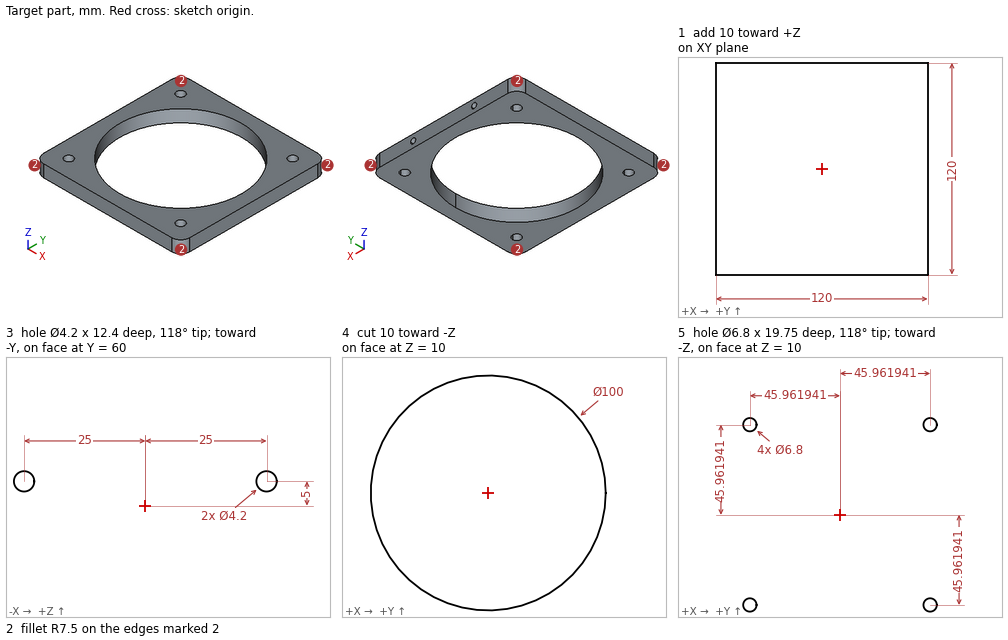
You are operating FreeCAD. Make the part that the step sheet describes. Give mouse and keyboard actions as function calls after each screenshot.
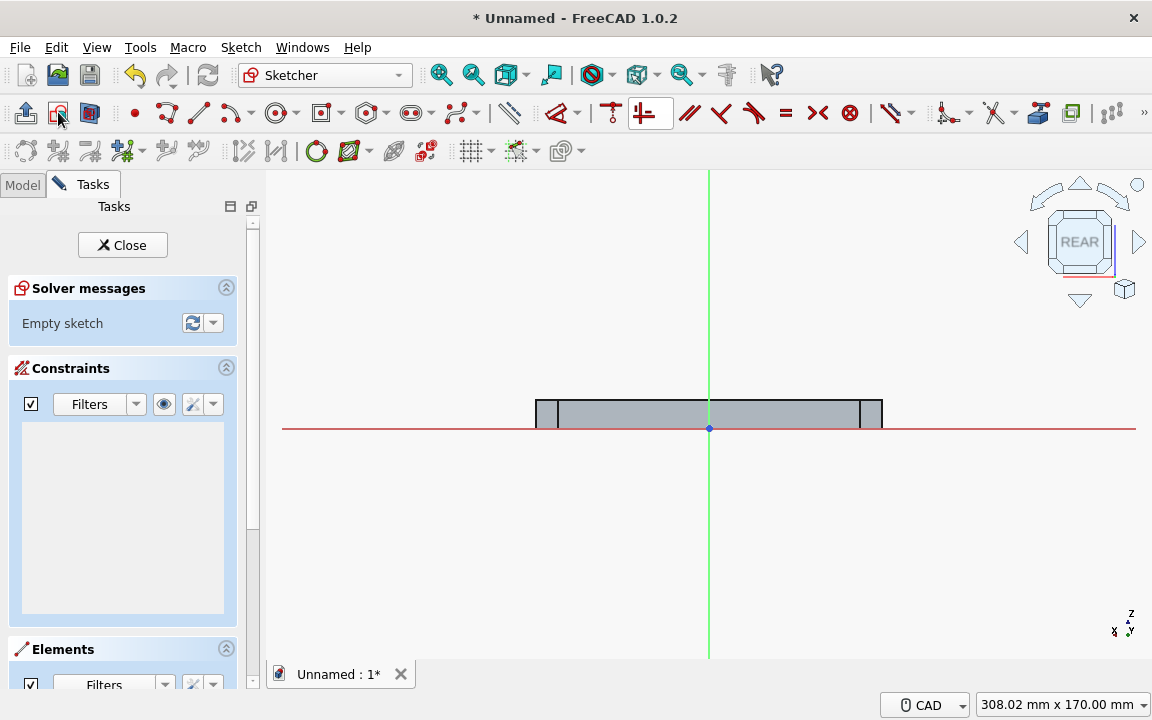
scroll(739, 420, up, 6)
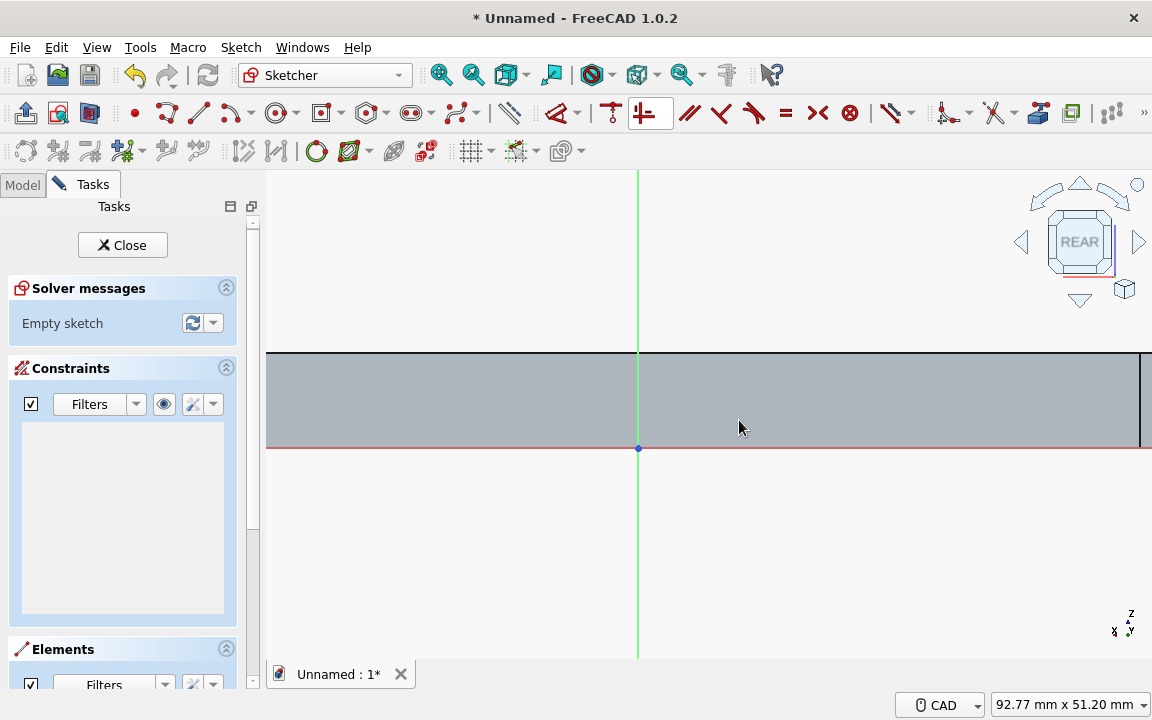
click(276, 114)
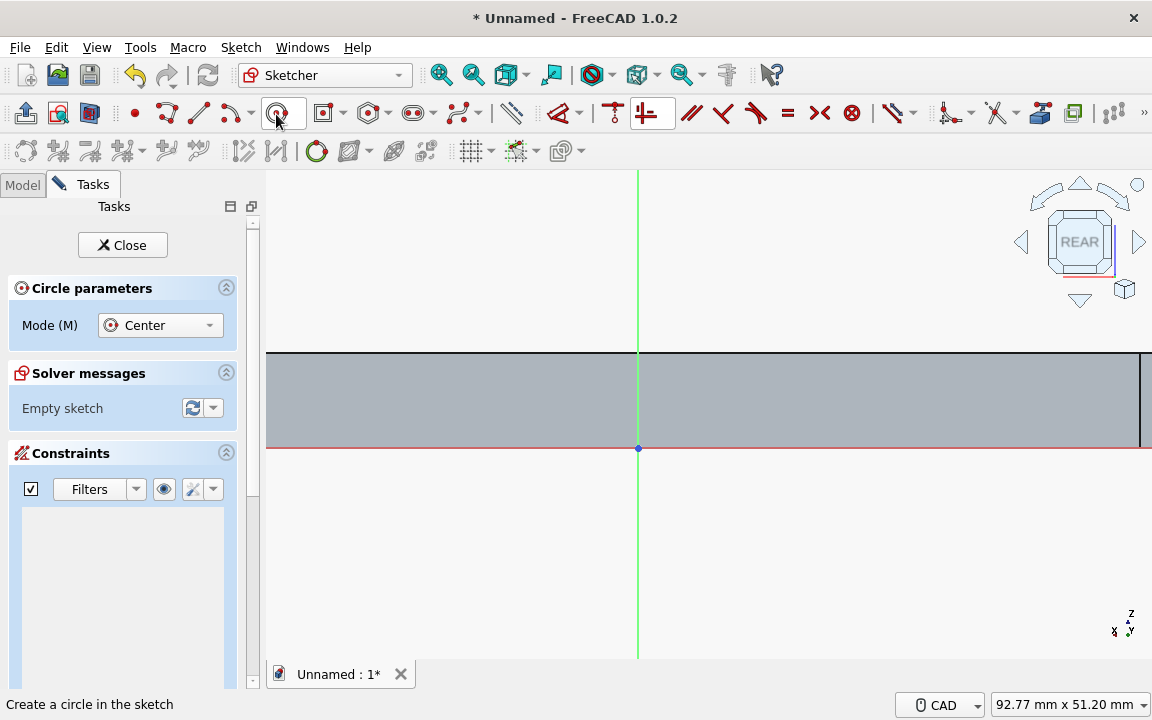
click(877, 401)
click(891, 386)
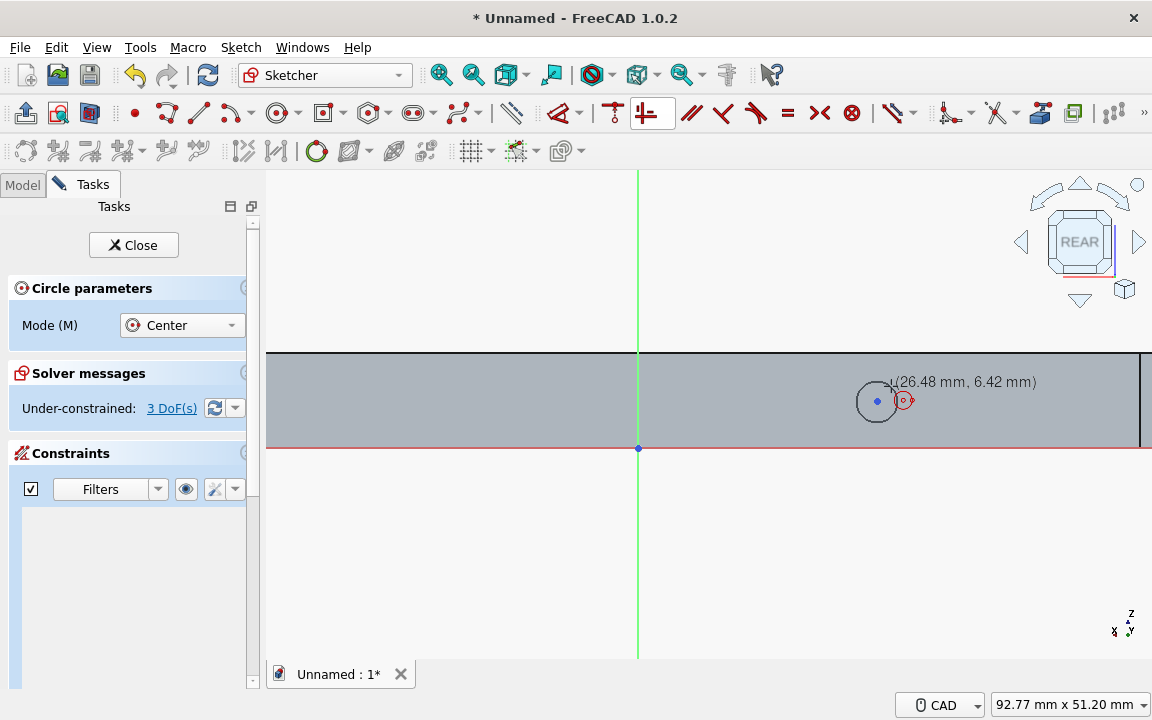
click(399, 401)
click(414, 386)
key(Escape)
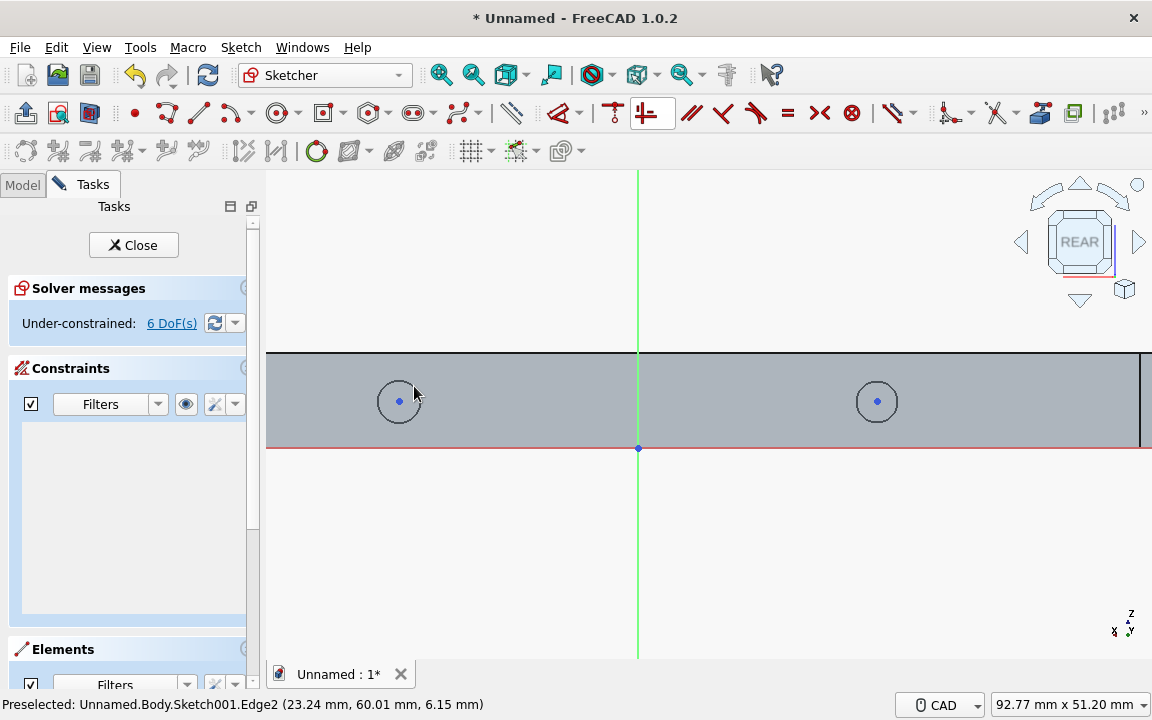
click(891, 387)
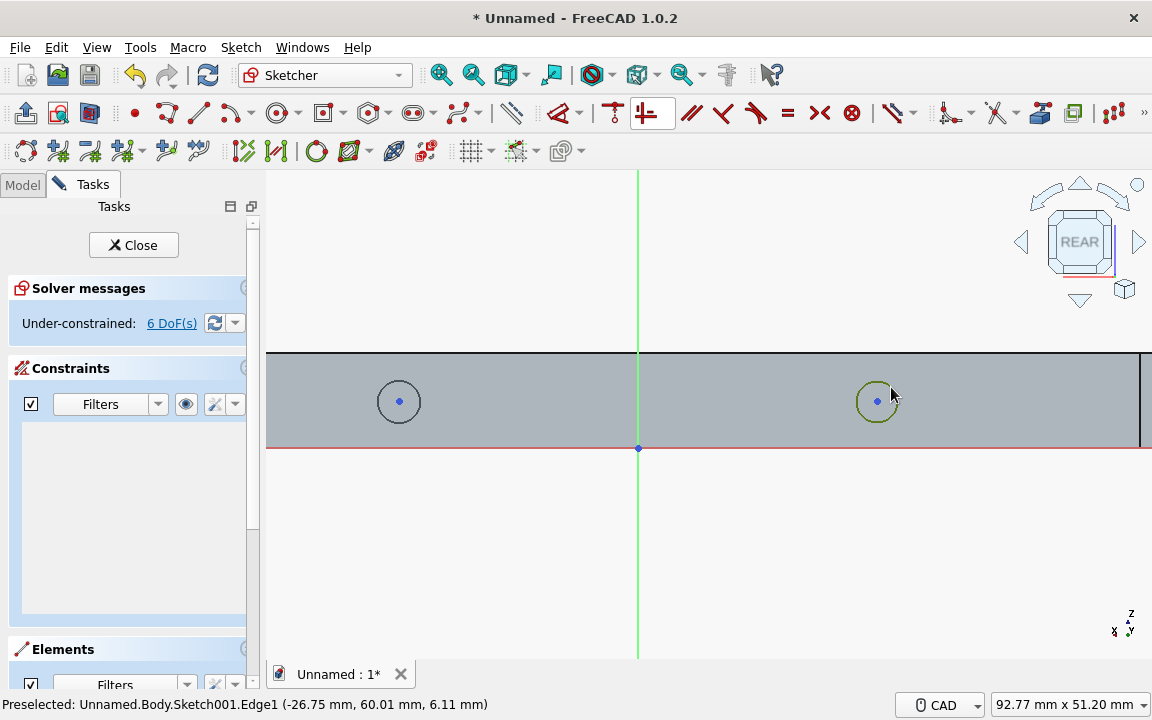
click(414, 387)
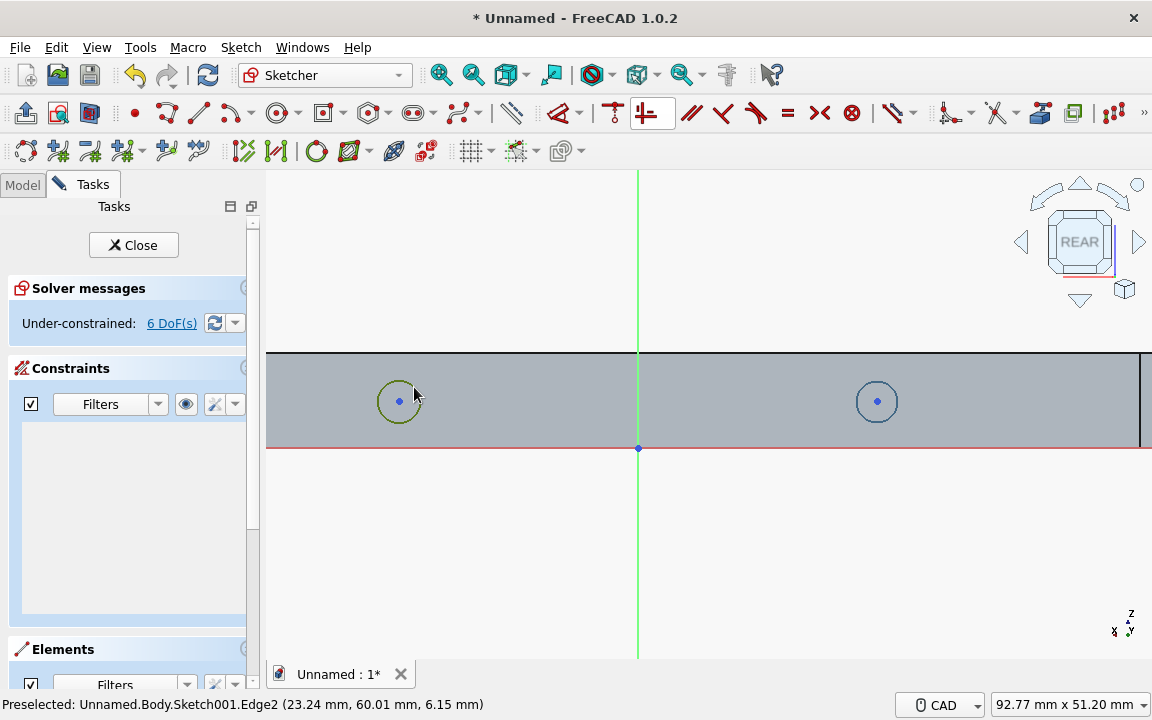
click(788, 114)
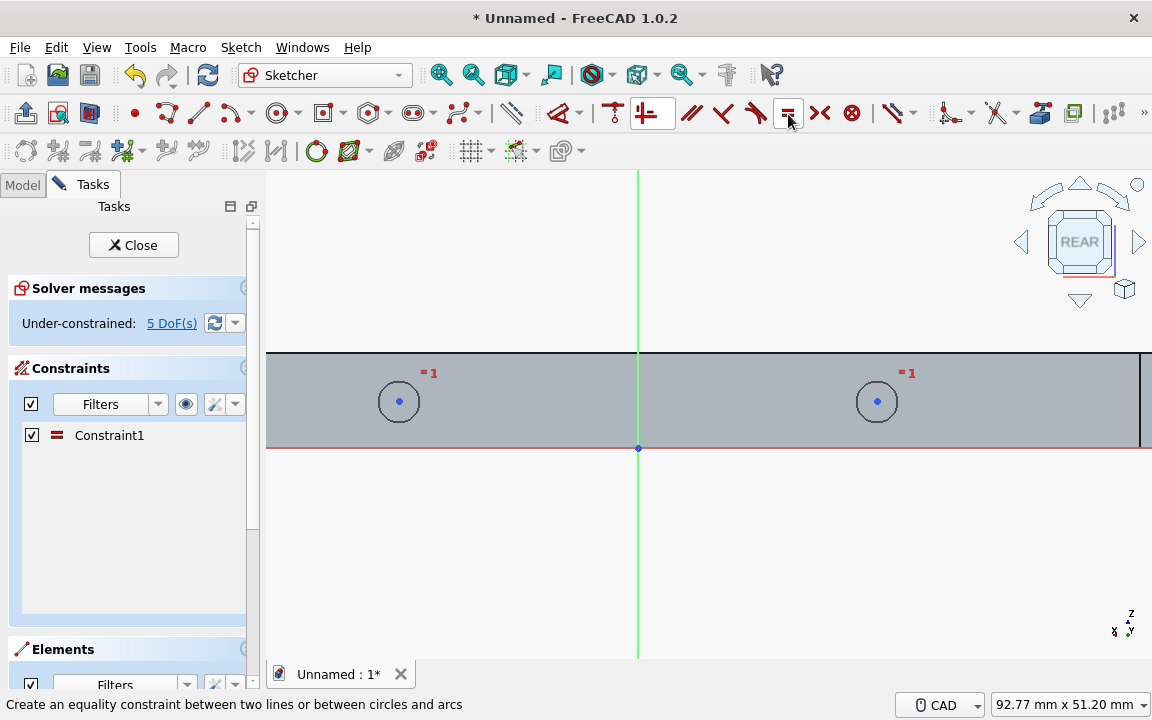
click(877, 402)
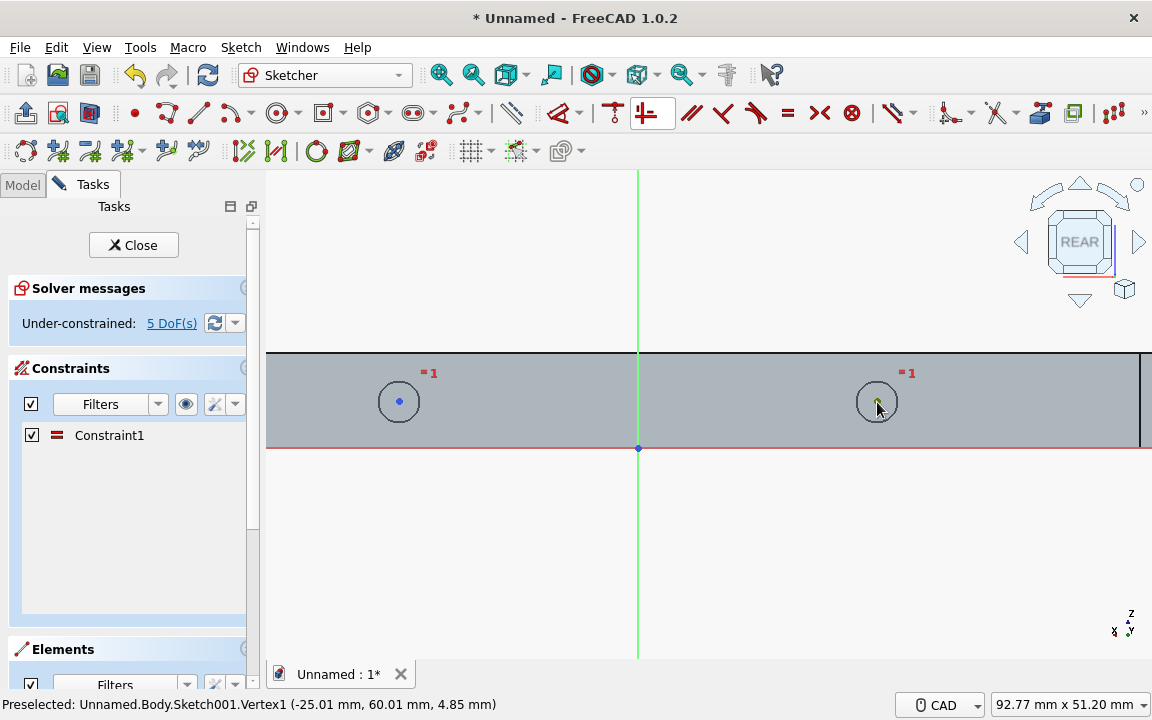
click(399, 402)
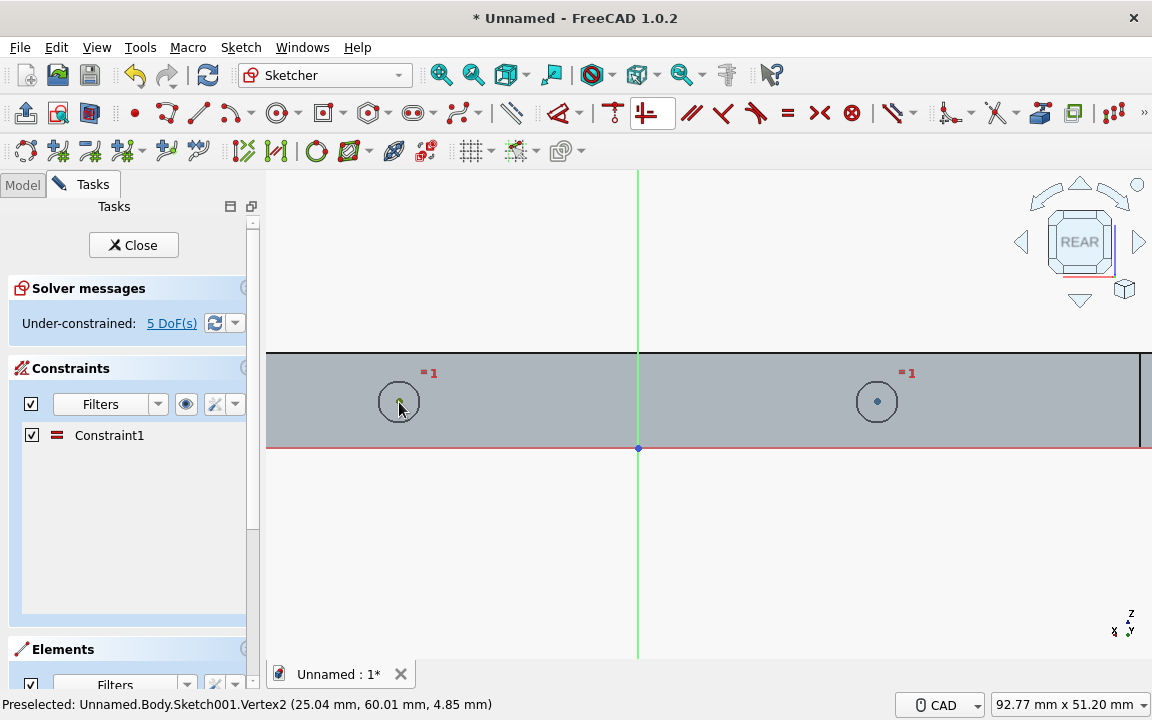
key(h)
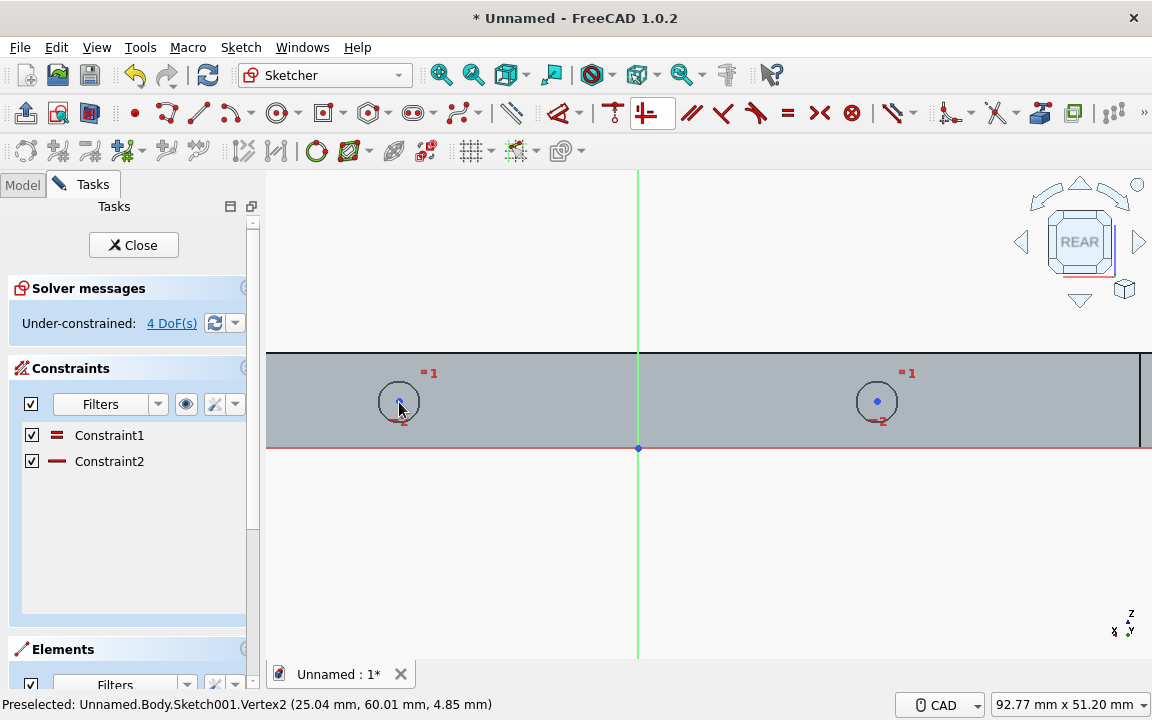
click(558, 114)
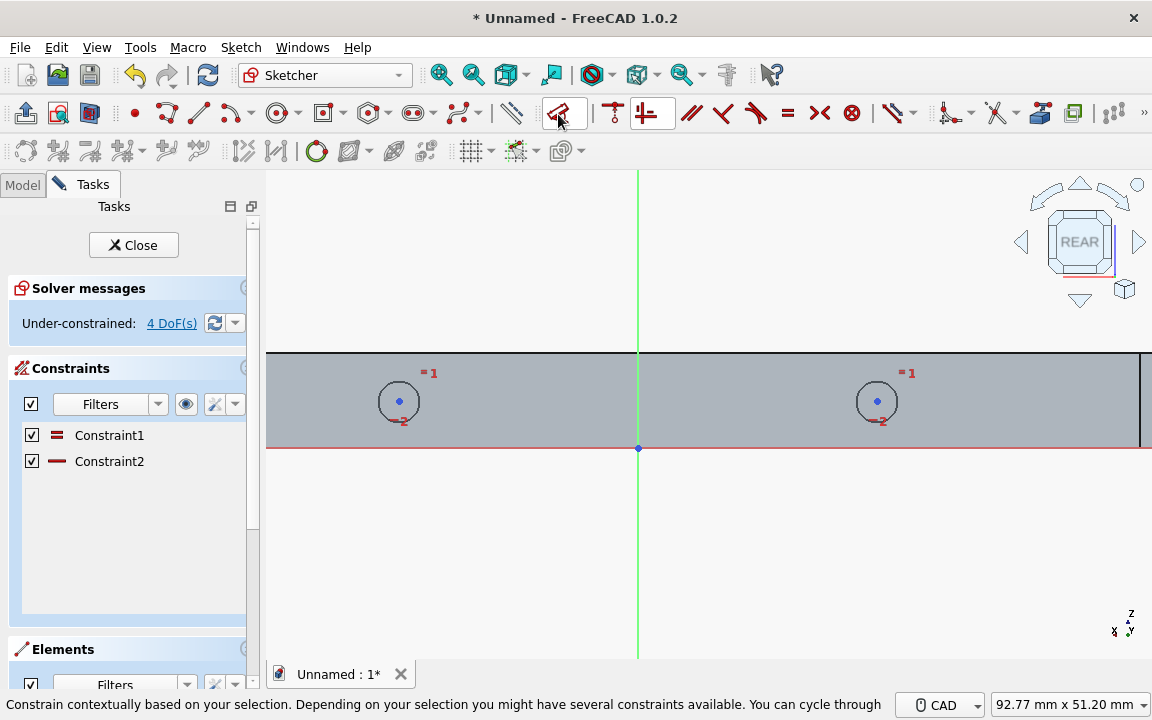
click(891, 387)
click(913, 364)